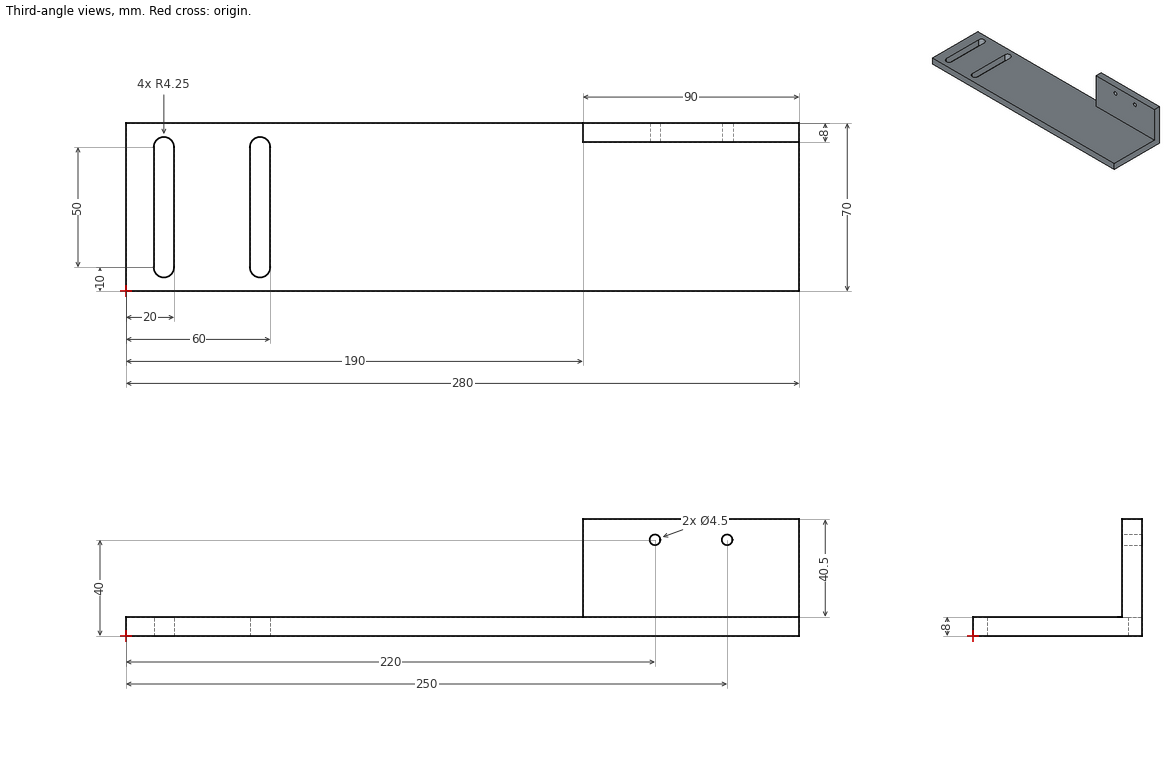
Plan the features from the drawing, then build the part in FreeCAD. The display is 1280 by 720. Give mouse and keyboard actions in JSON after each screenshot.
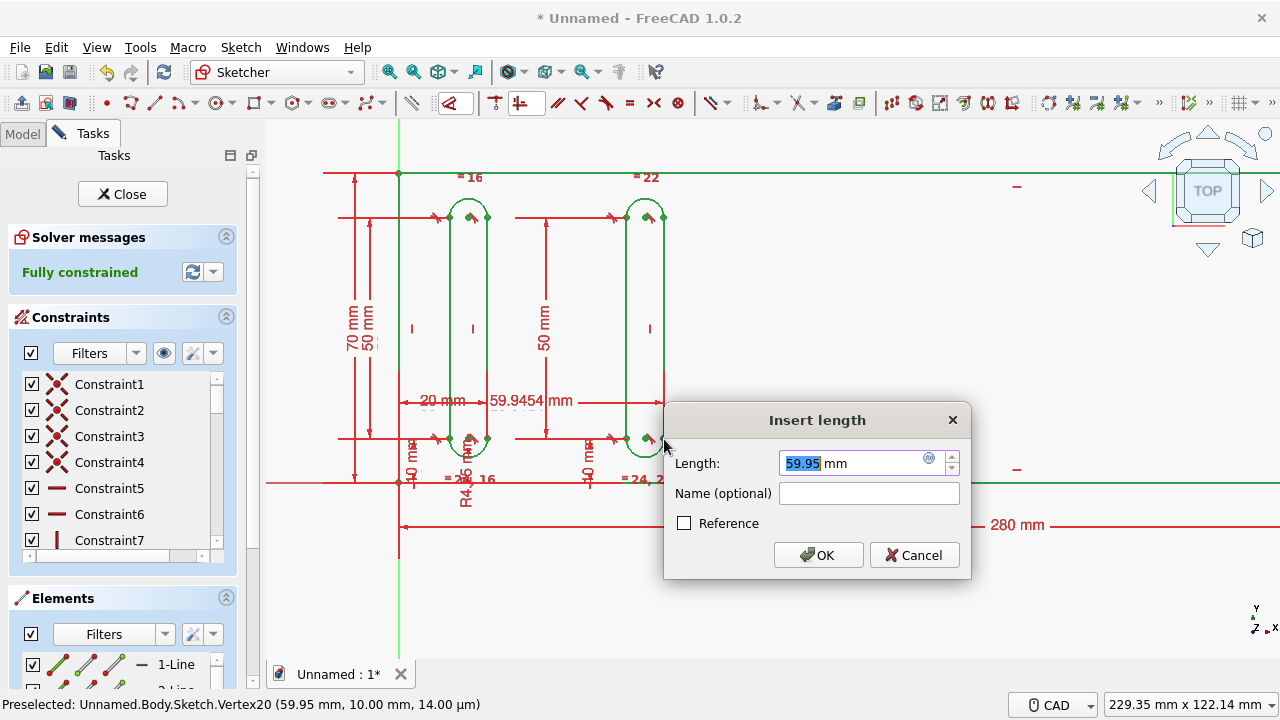
{"action": "type", "text": "60"}
{"action": "key", "text": "Return"}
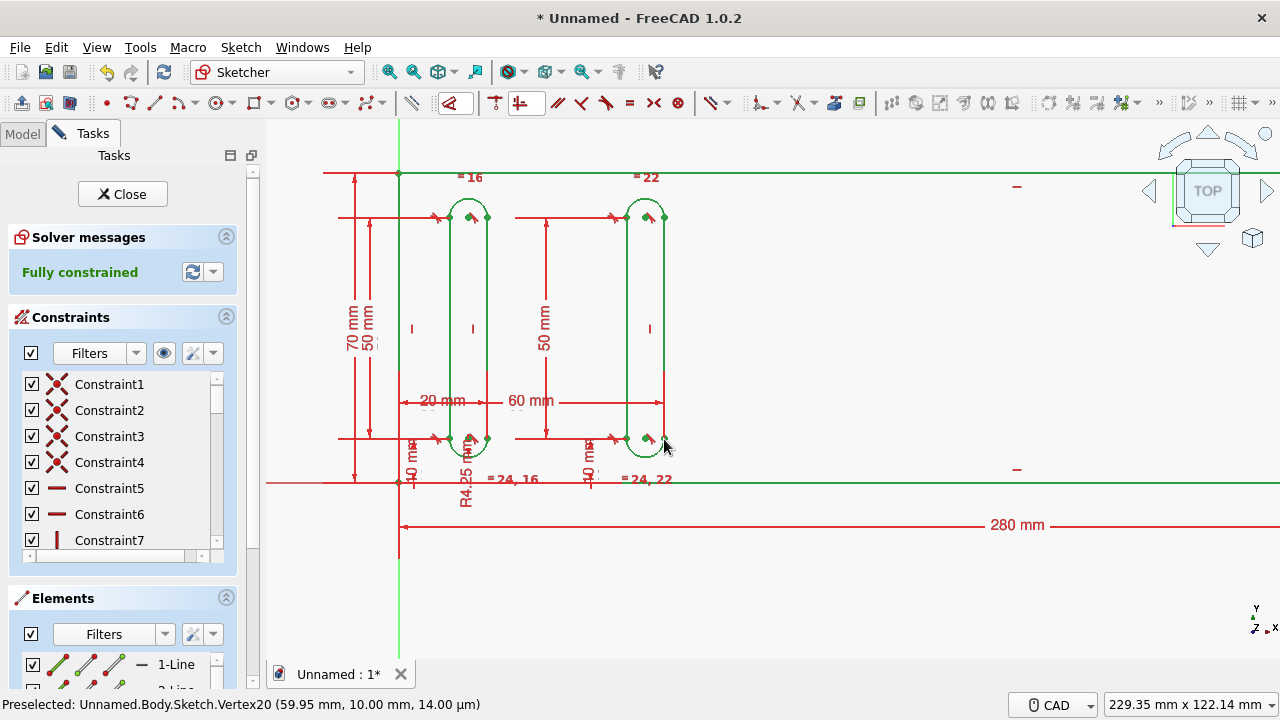
{"action": "left_click", "coordinate": [123, 194]}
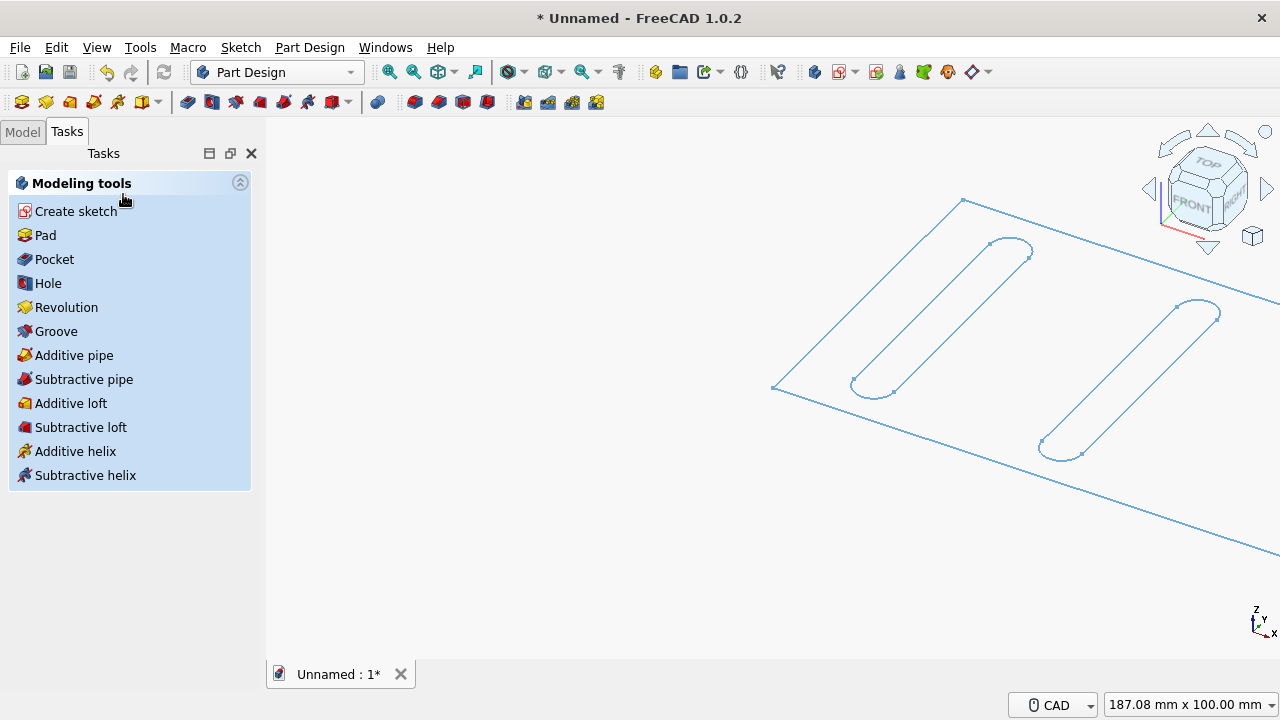
{"action": "left_click", "coordinate": [22, 102]}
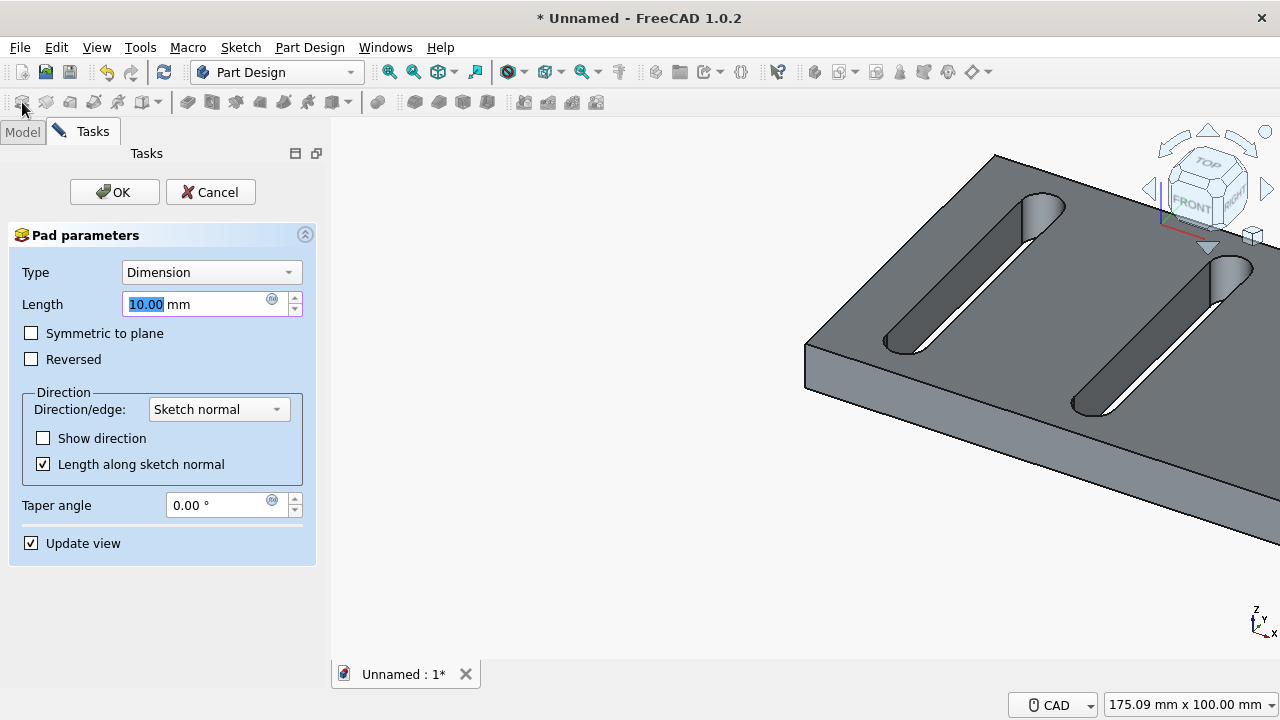
{"action": "type", "text": "8"}
{"action": "key", "text": "Tab"}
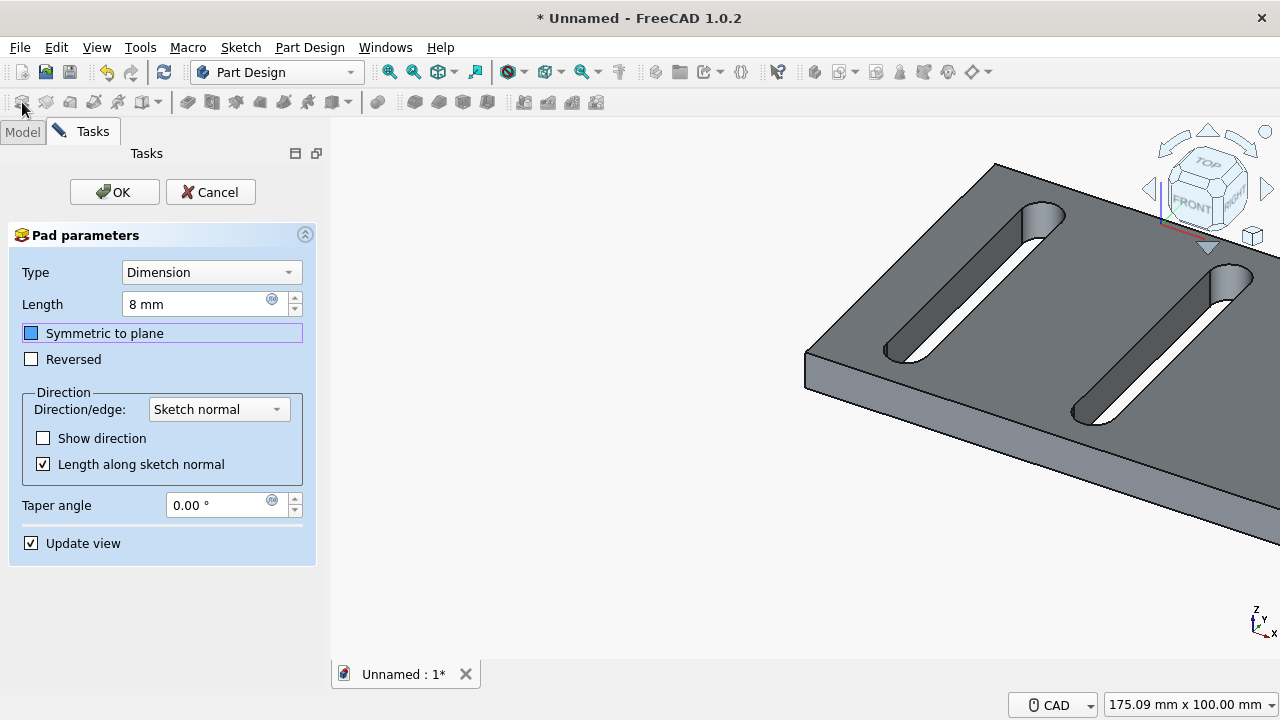
{"action": "left_click", "coordinate": [115, 192]}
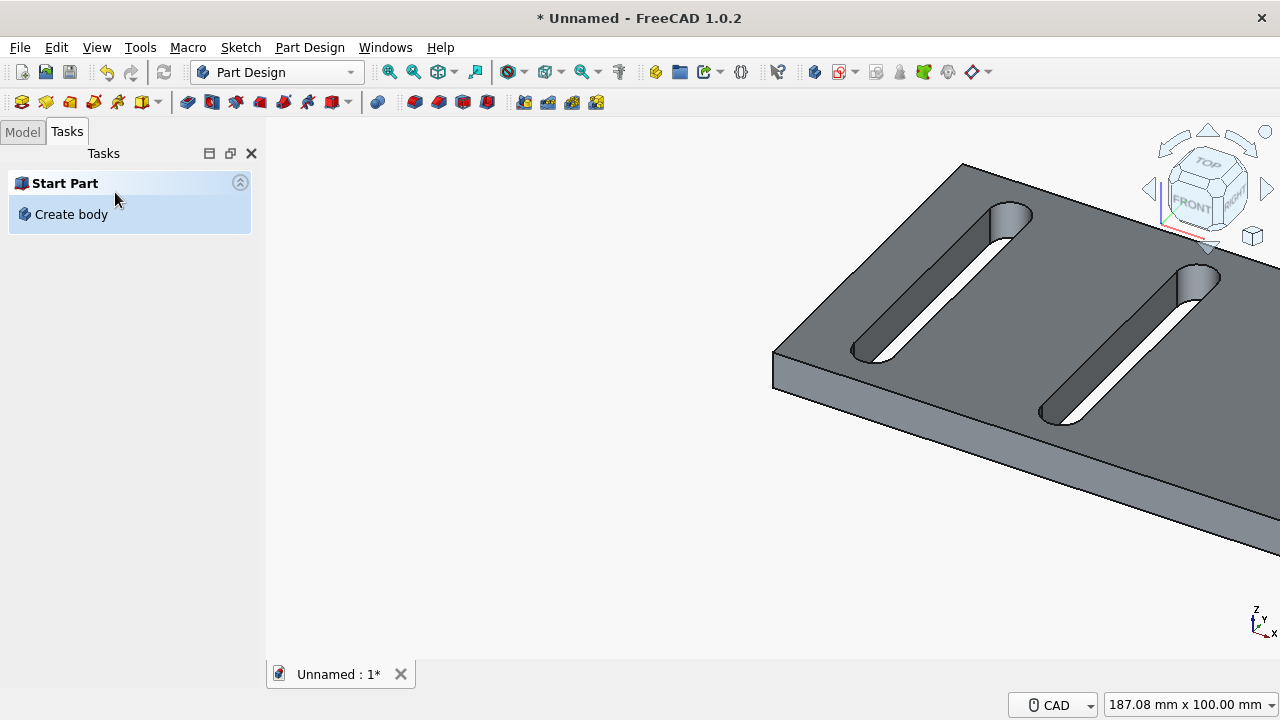
{"action": "key", "text": "v f"}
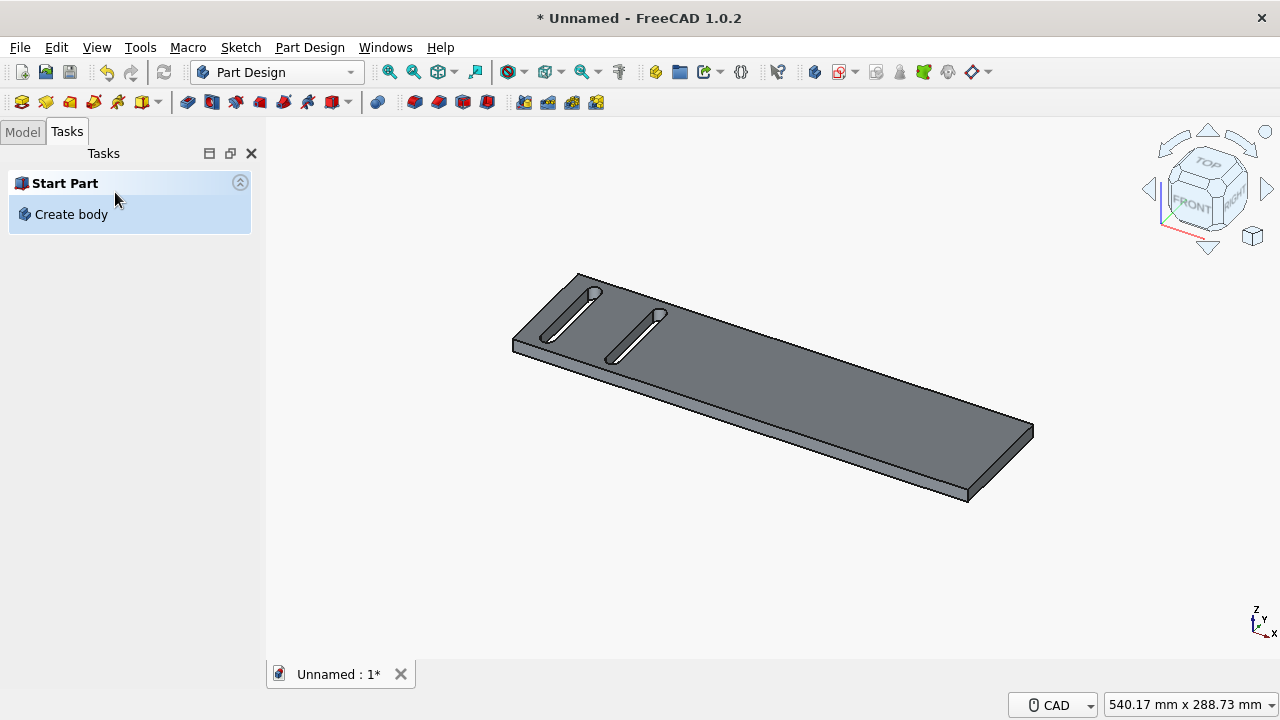
{"action": "left_click", "coordinate": [903, 424]}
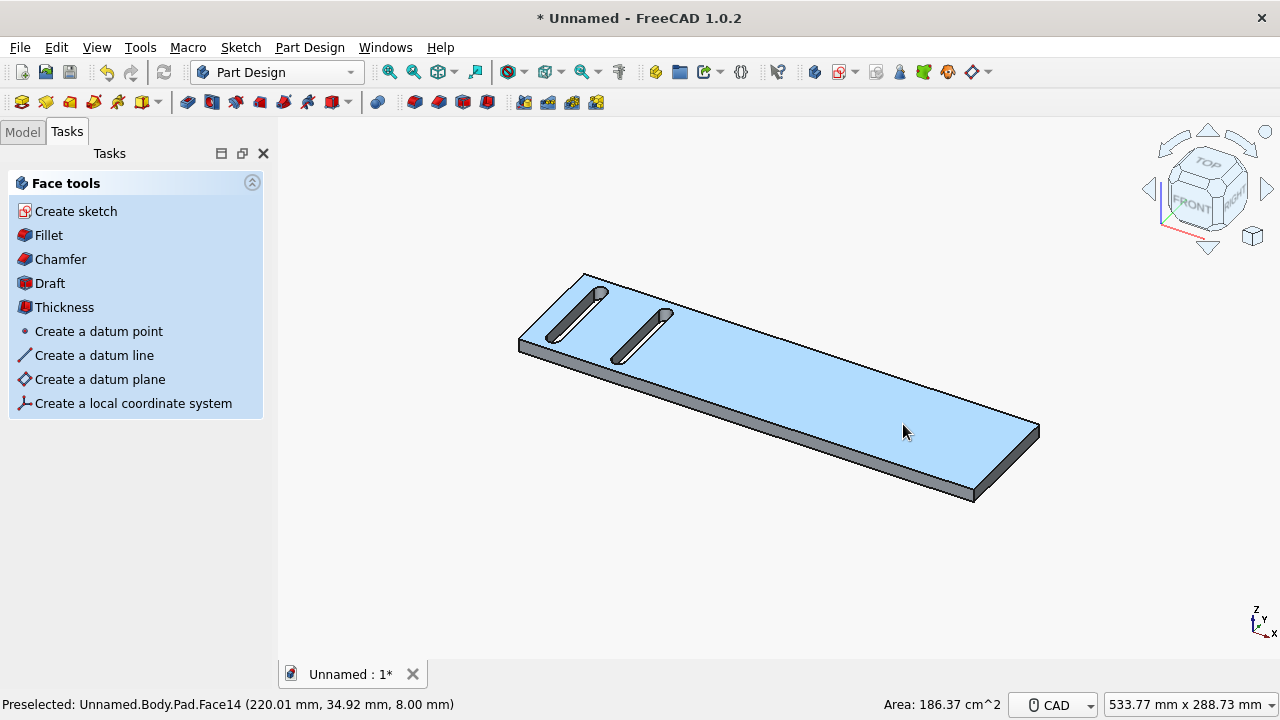
{"action": "left_click", "coordinate": [840, 72]}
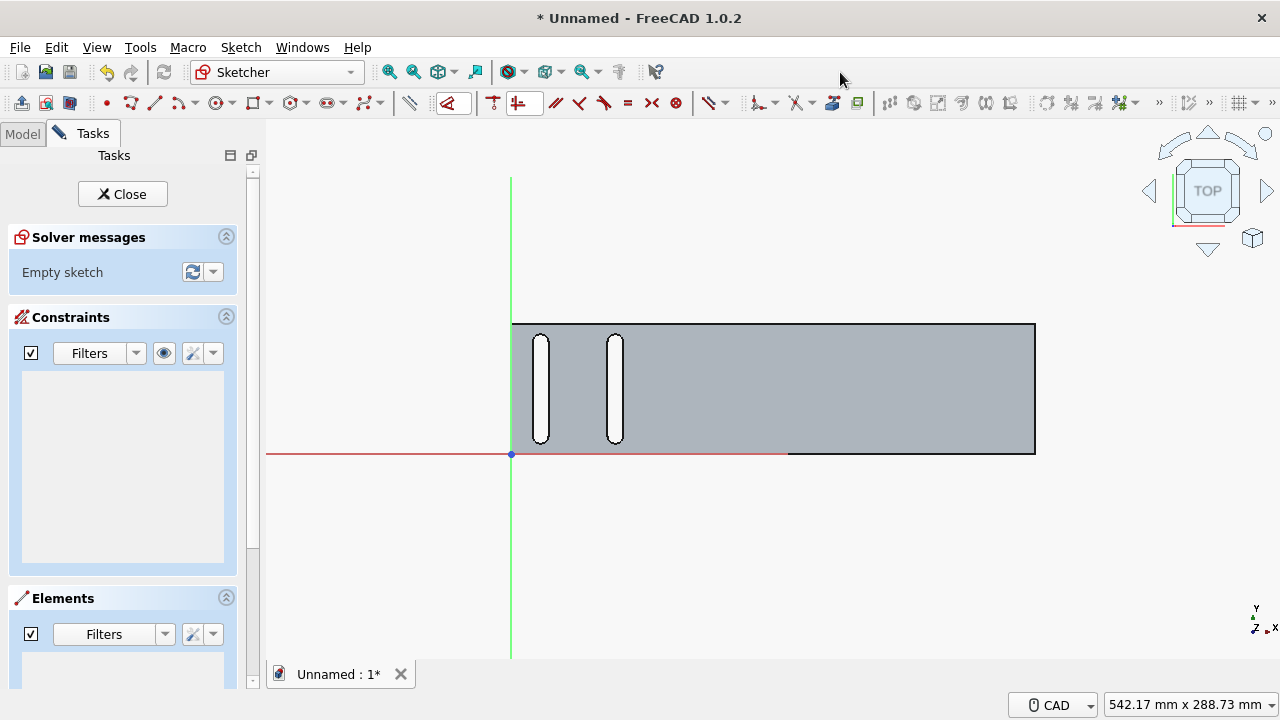
{"action": "scroll", "coordinate": [1057, 306], "scroll_direction": "up", "scroll_amount": 6}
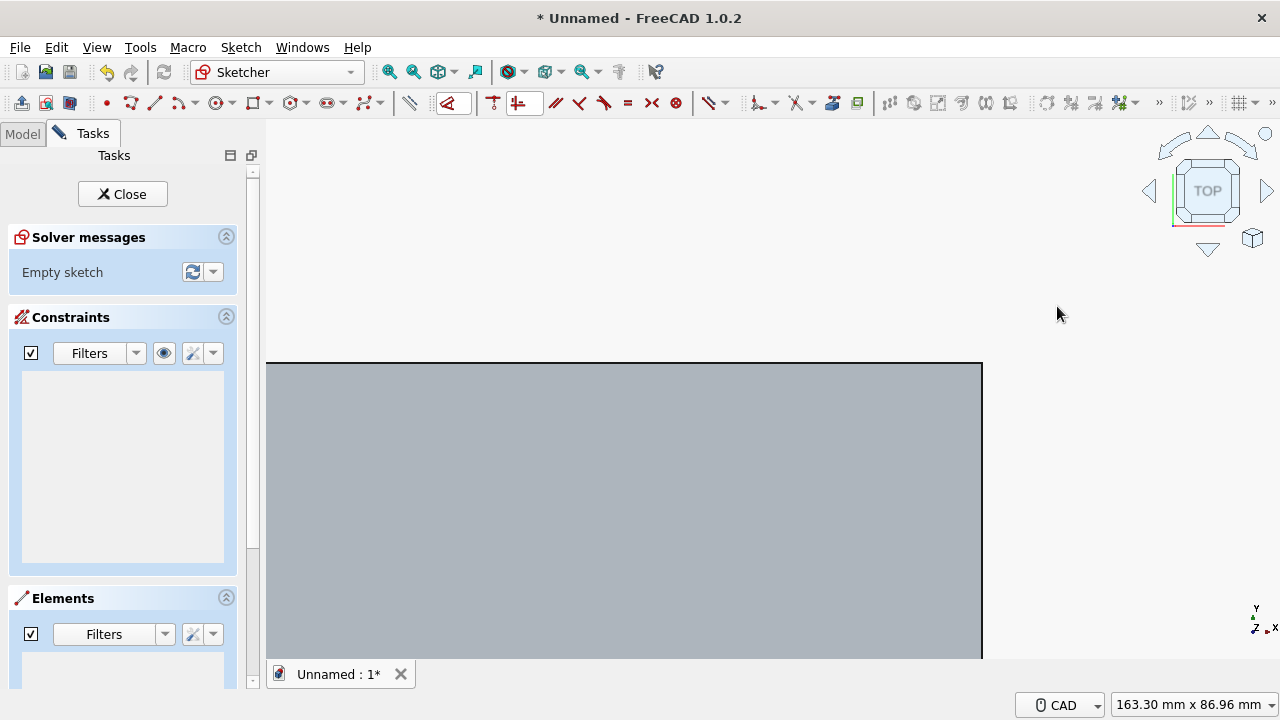
{"action": "left_click", "coordinate": [254, 104]}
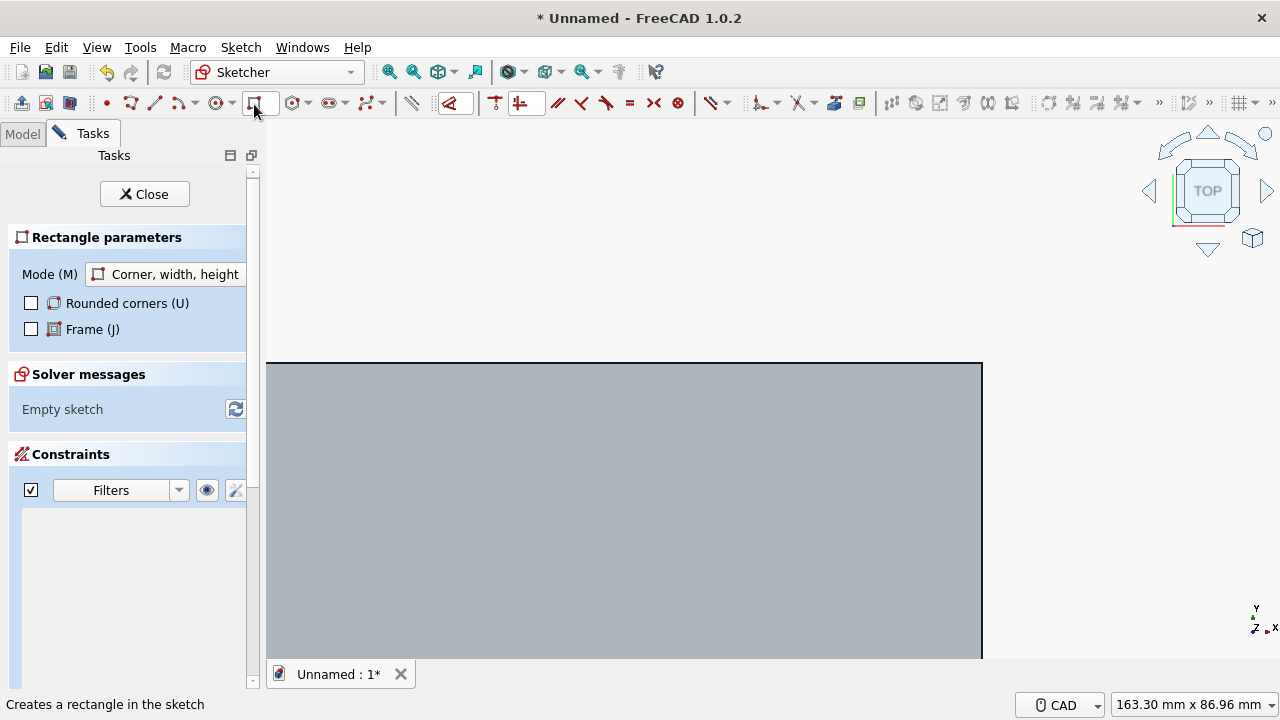
{"action": "left_click", "coordinate": [423, 363]}
{"action": "mouse_move", "coordinate": [982, 413]}